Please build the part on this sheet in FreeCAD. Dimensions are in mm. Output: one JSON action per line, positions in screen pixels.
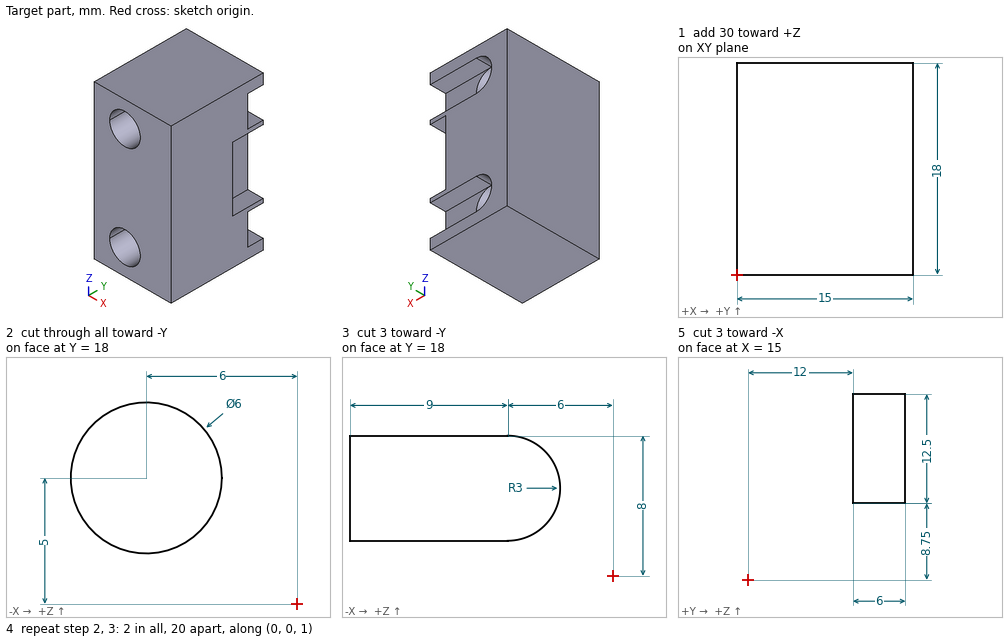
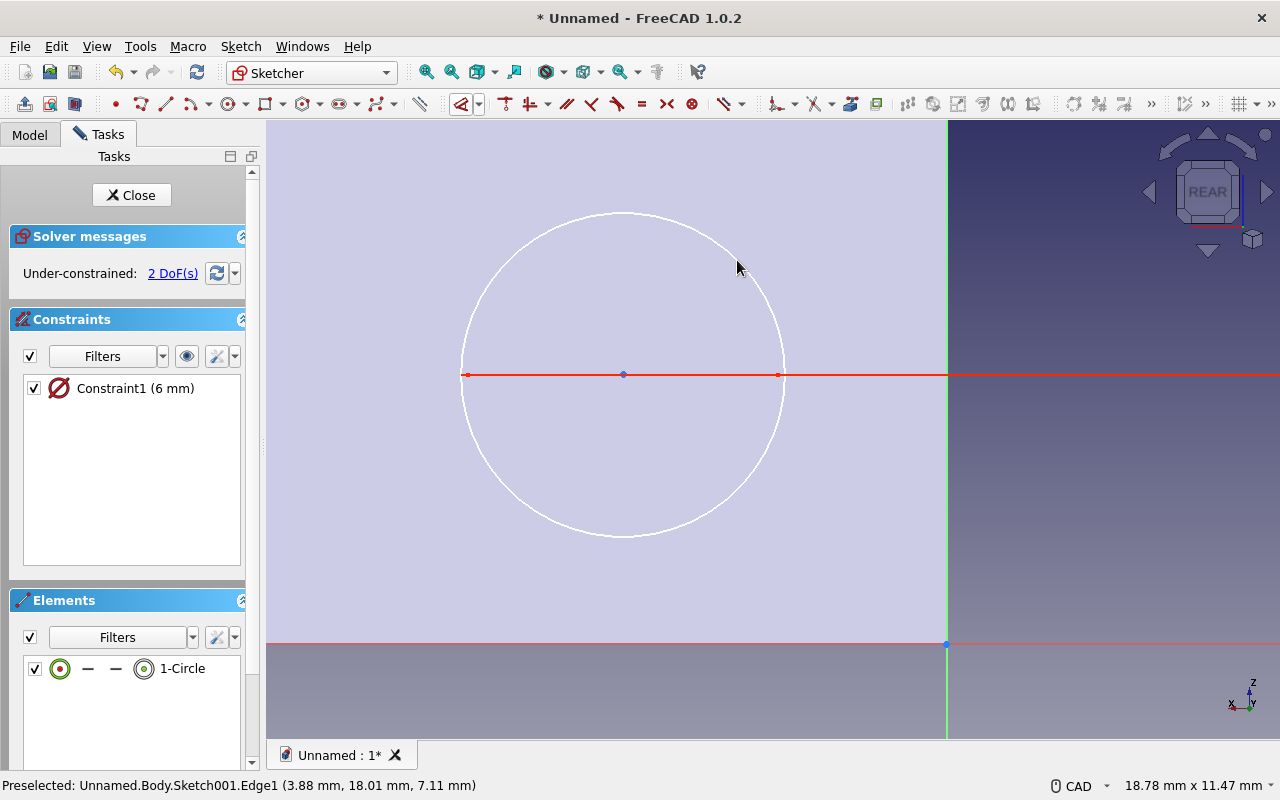
{"action": "left_click", "coordinate": [623, 375]}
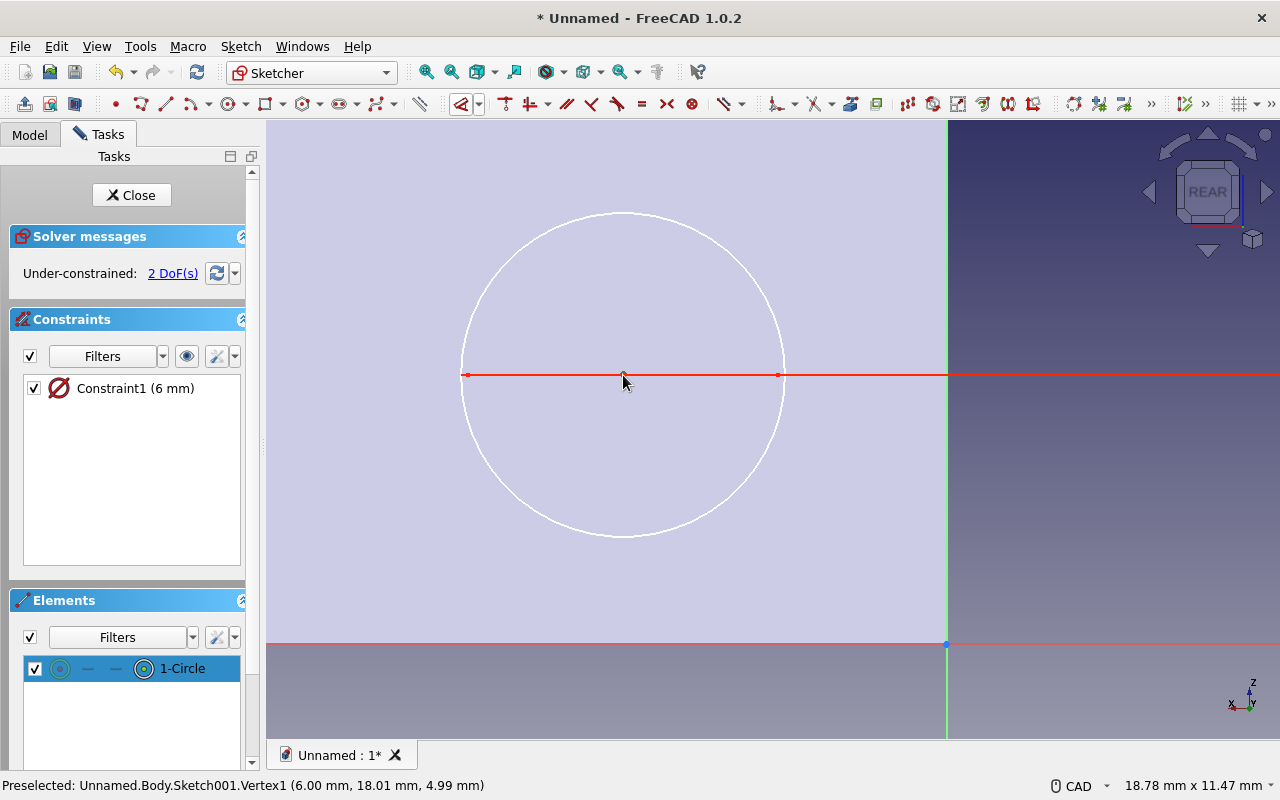
{"action": "key", "text": "l"}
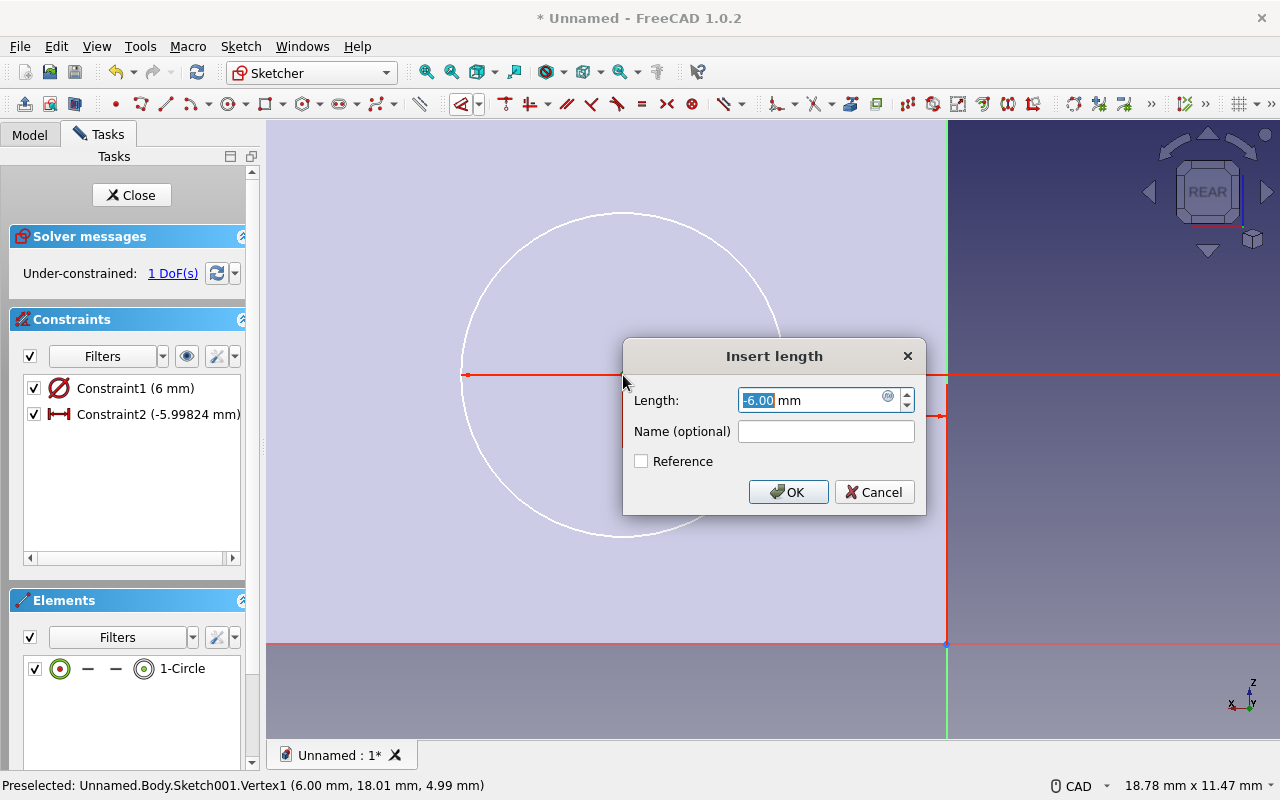
{"action": "type", "text": "-6"}
{"action": "key", "text": "Return"}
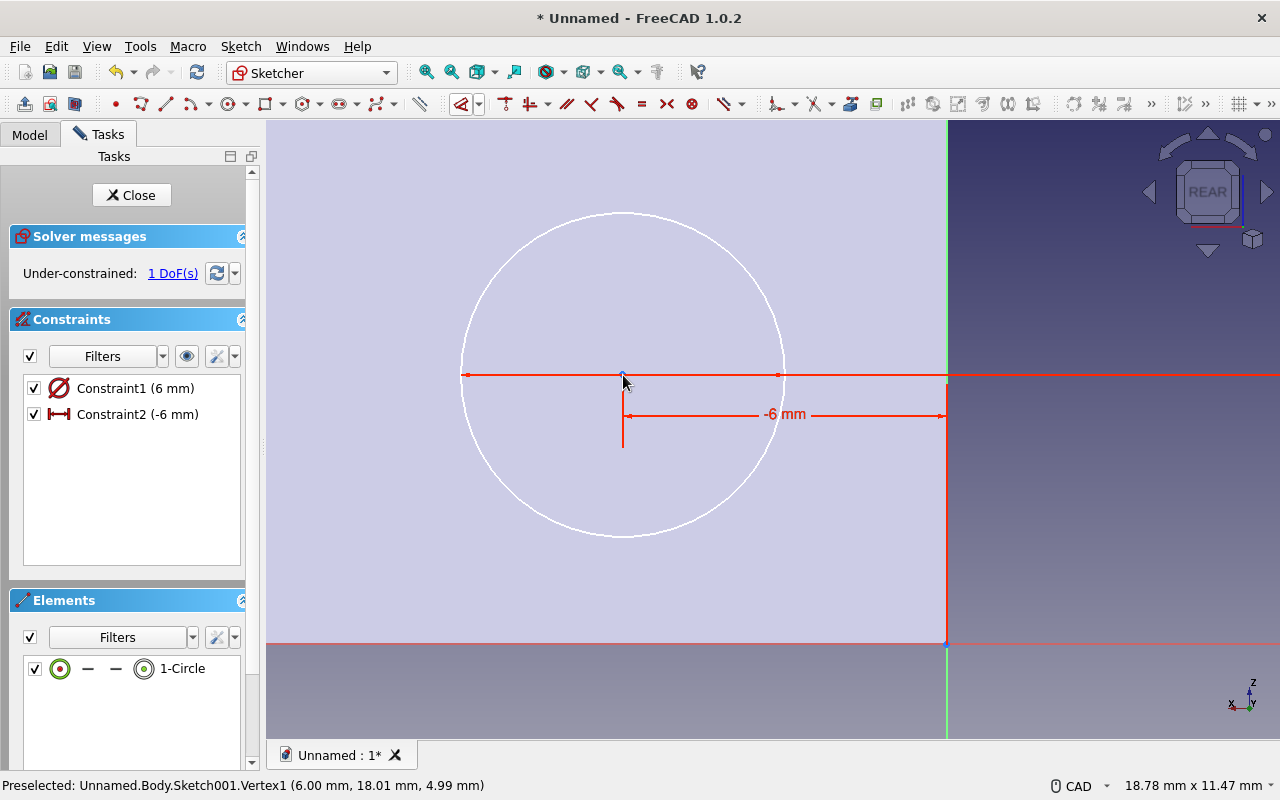
{"action": "left_click", "coordinate": [623, 375]}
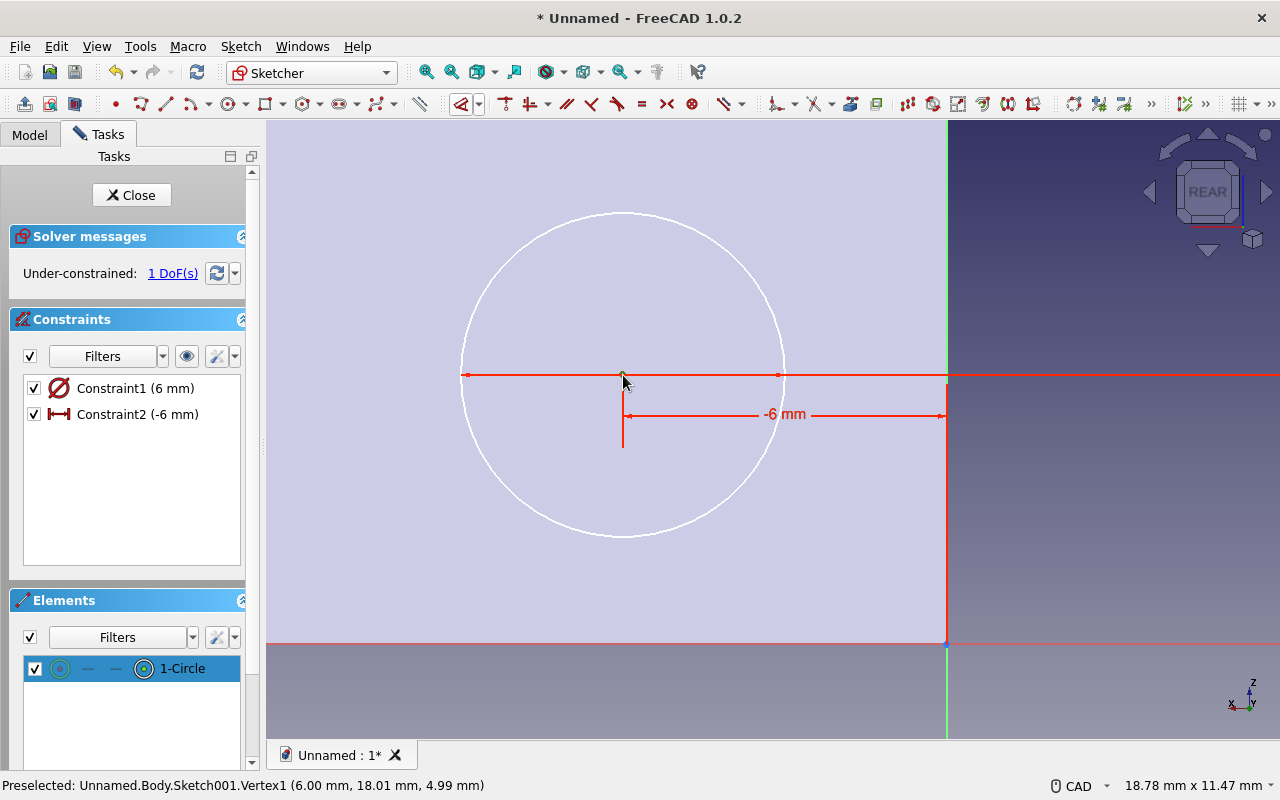
{"action": "key", "text": "i"}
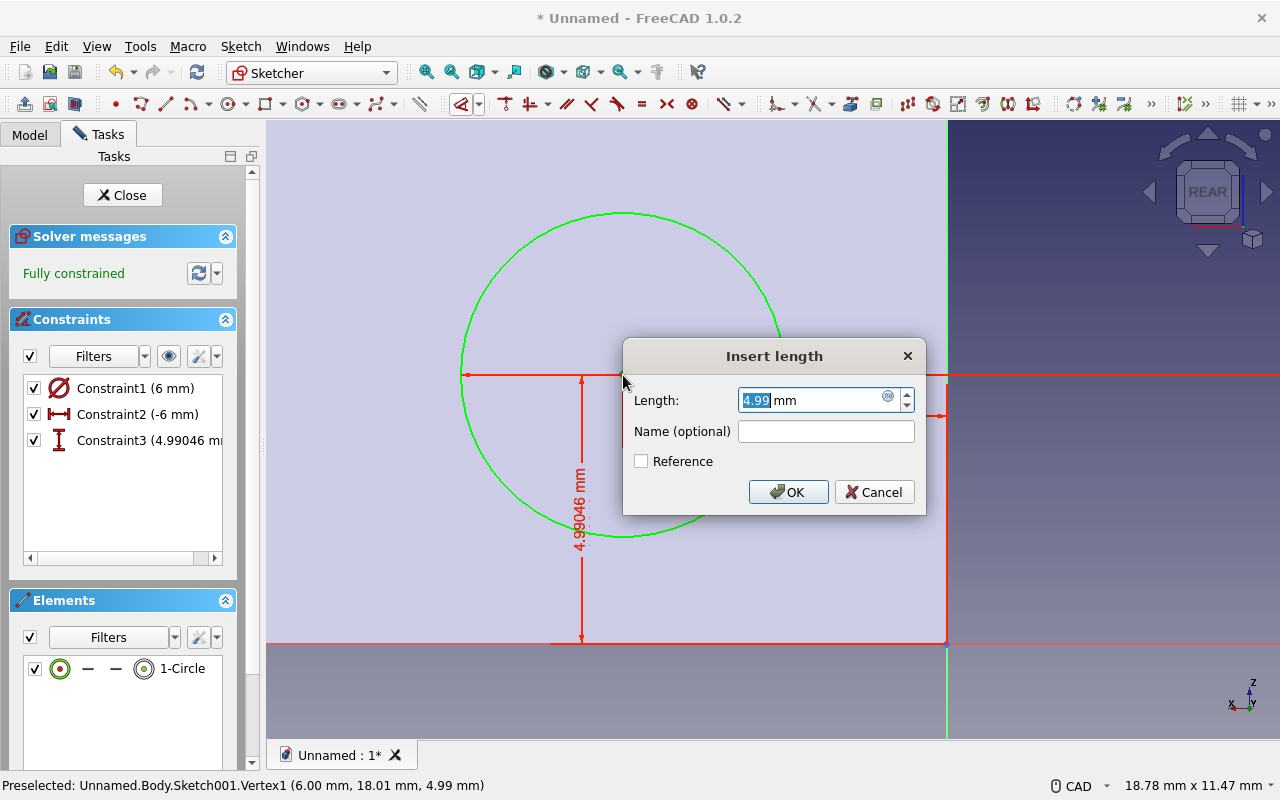
{"action": "type", "text": "5"}
{"action": "key", "text": "Return"}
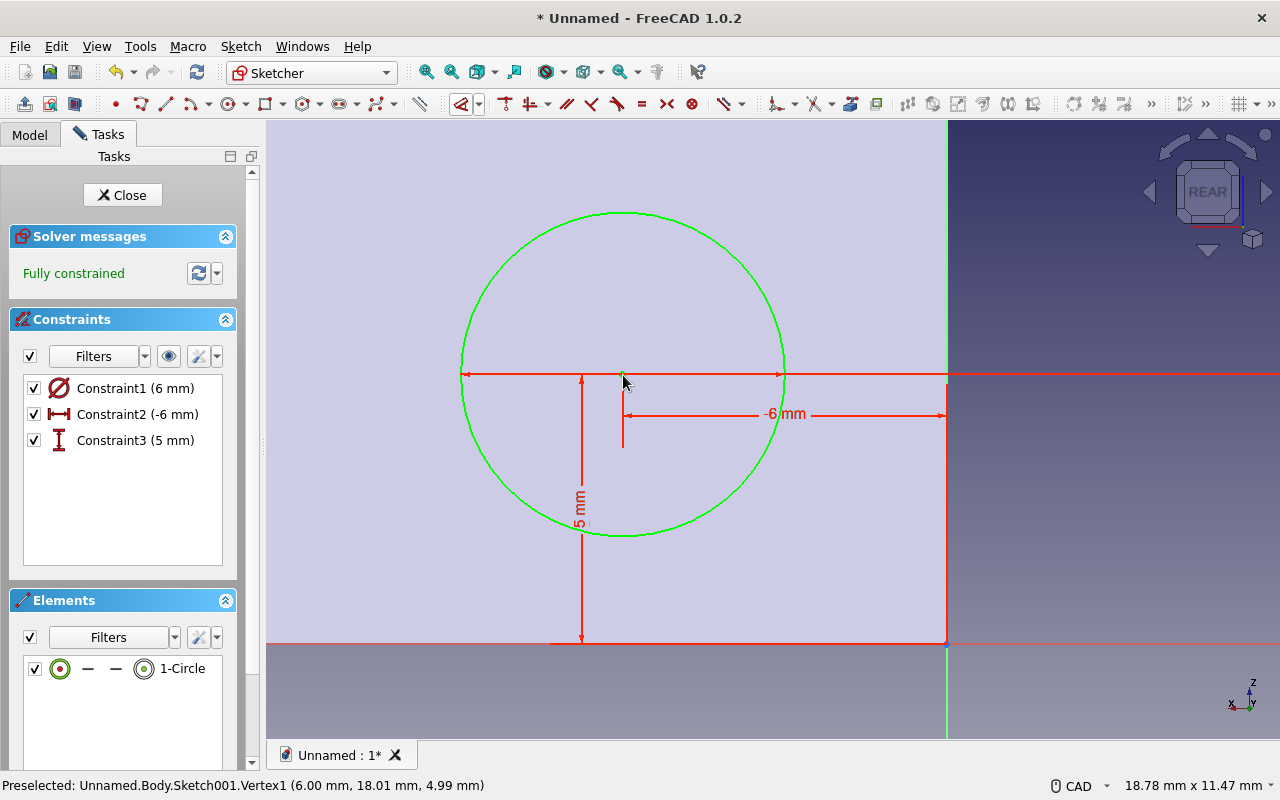
{"action": "left_click", "coordinate": [123, 195]}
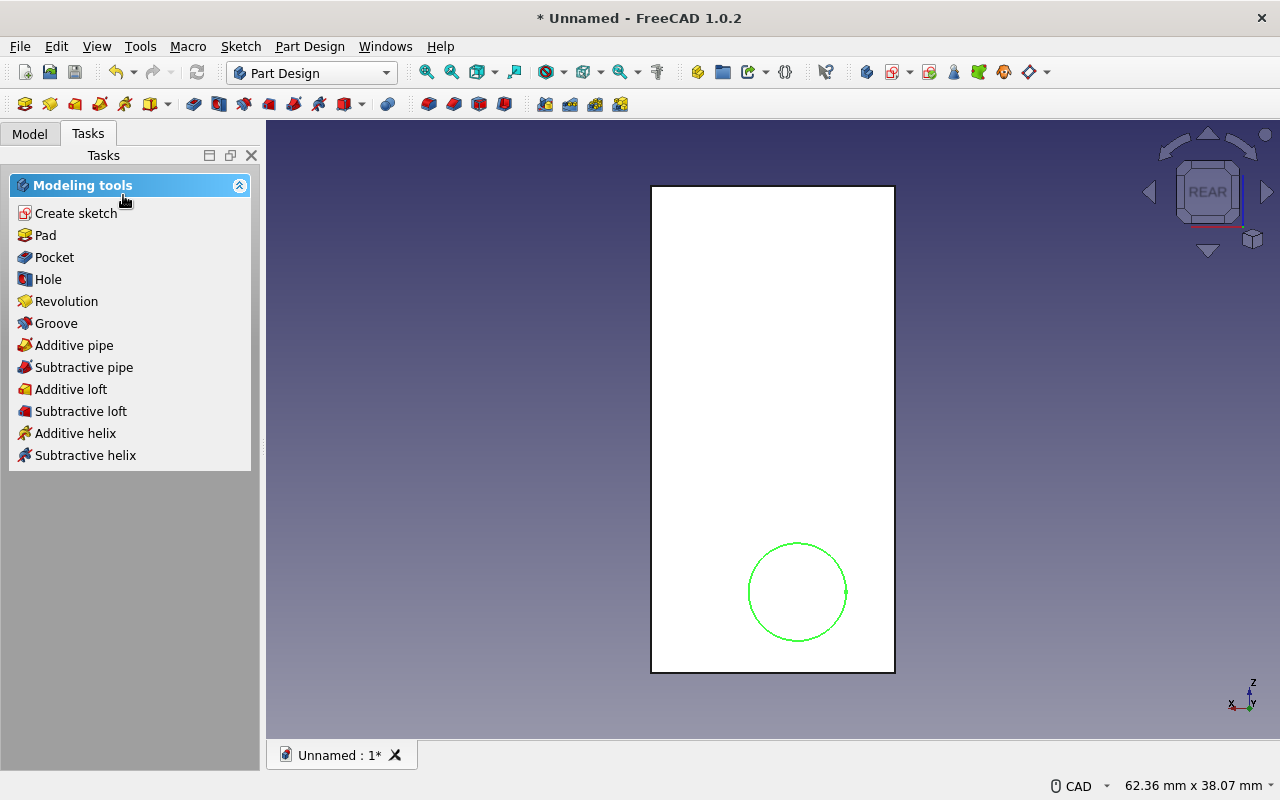
{"action": "left_click", "coordinate": [194, 104]}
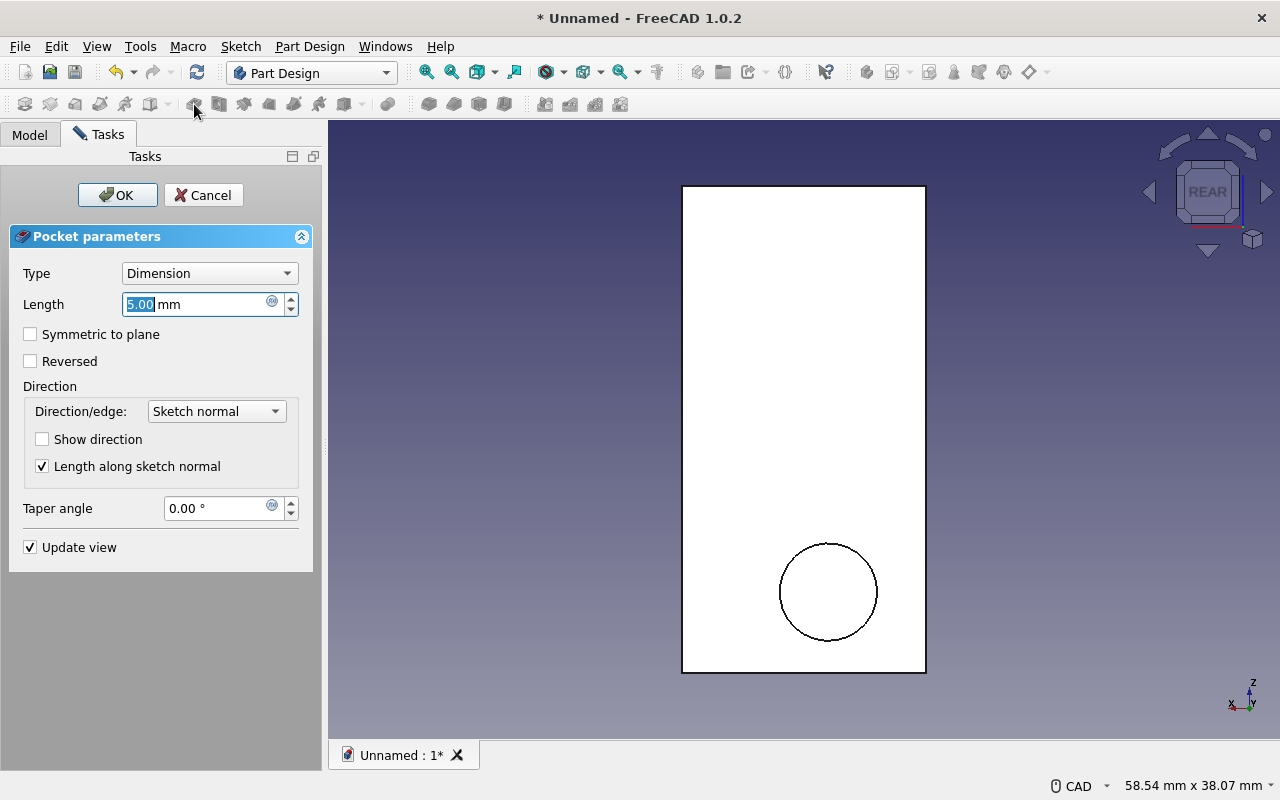
{"action": "left_click", "coordinate": [210, 274]}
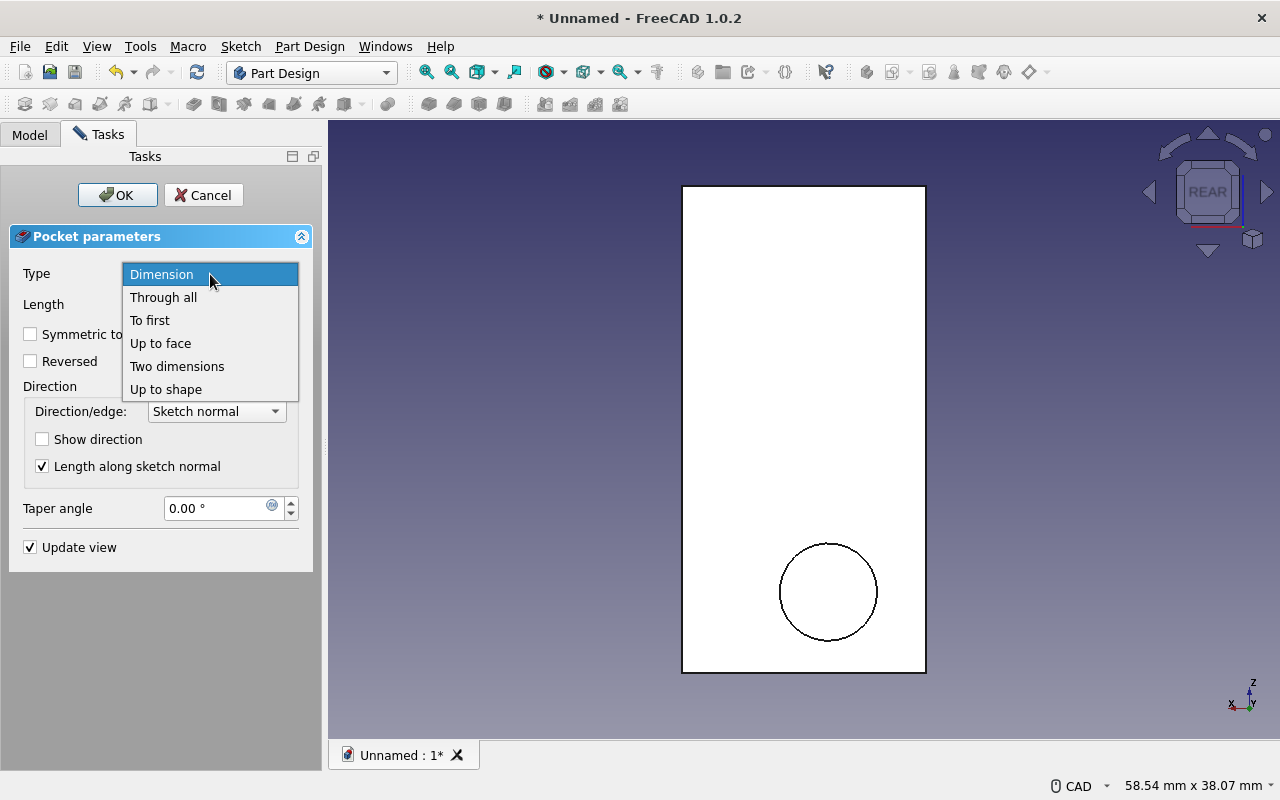
{"action": "left_click", "coordinate": [208, 298]}